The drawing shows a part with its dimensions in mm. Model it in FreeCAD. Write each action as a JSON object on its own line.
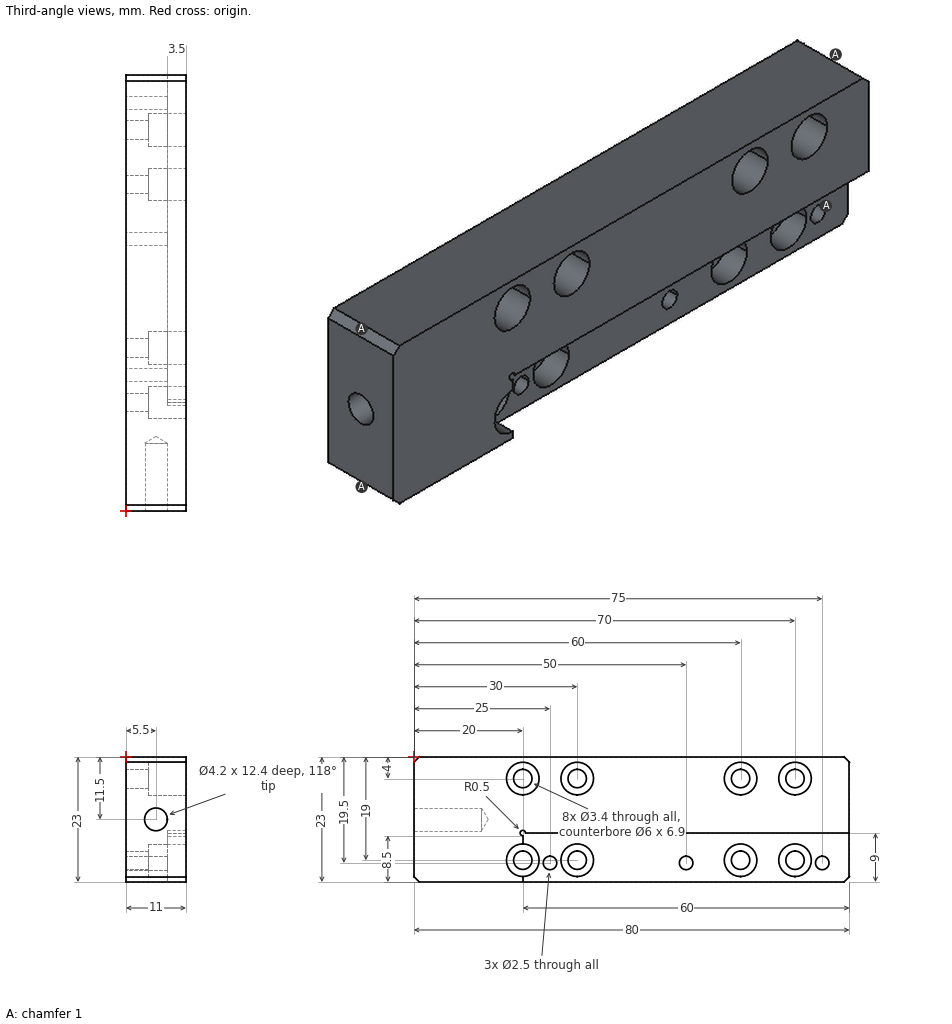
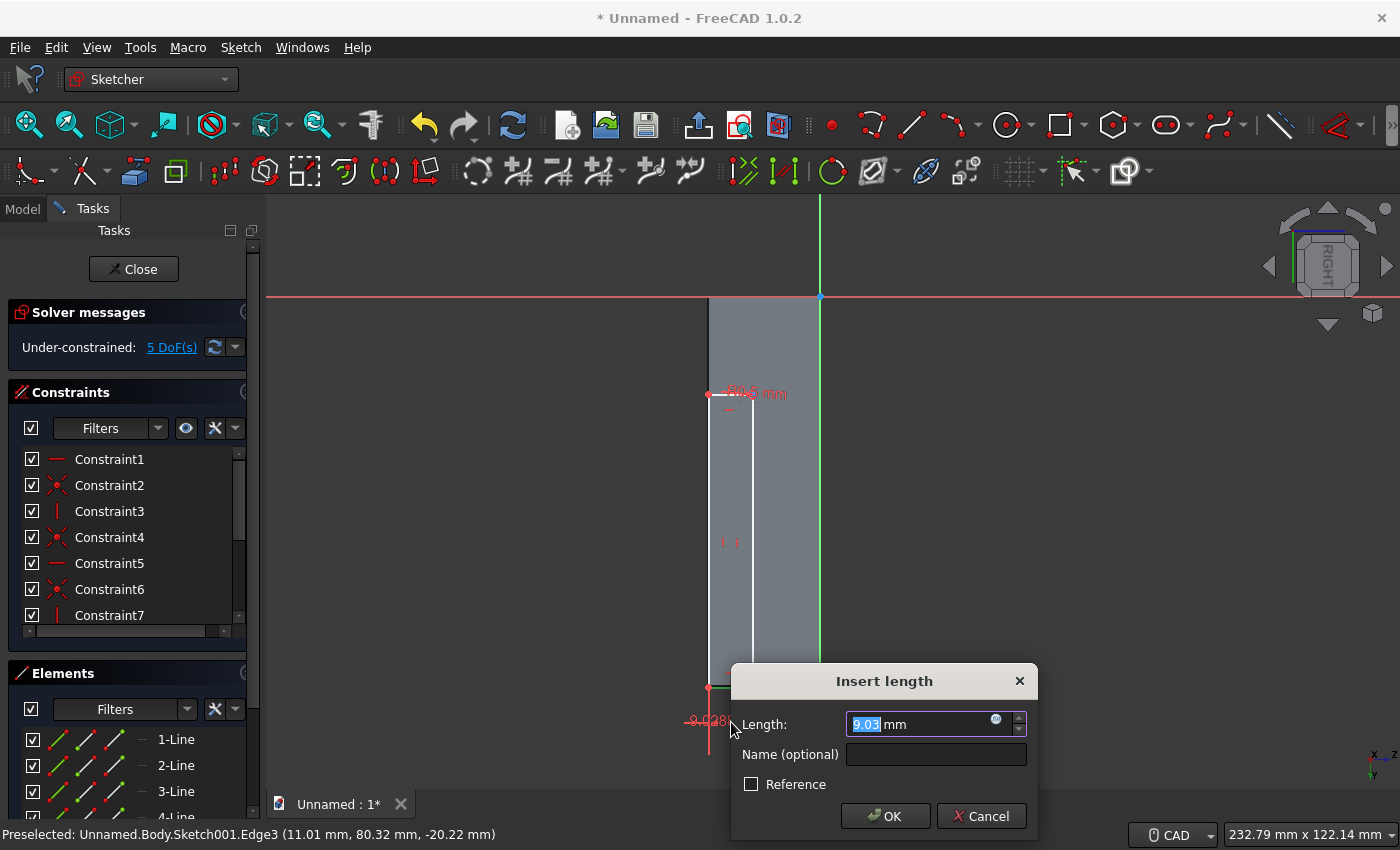
{"action": "type", "text": "9"}
{"action": "key", "text": "Return"}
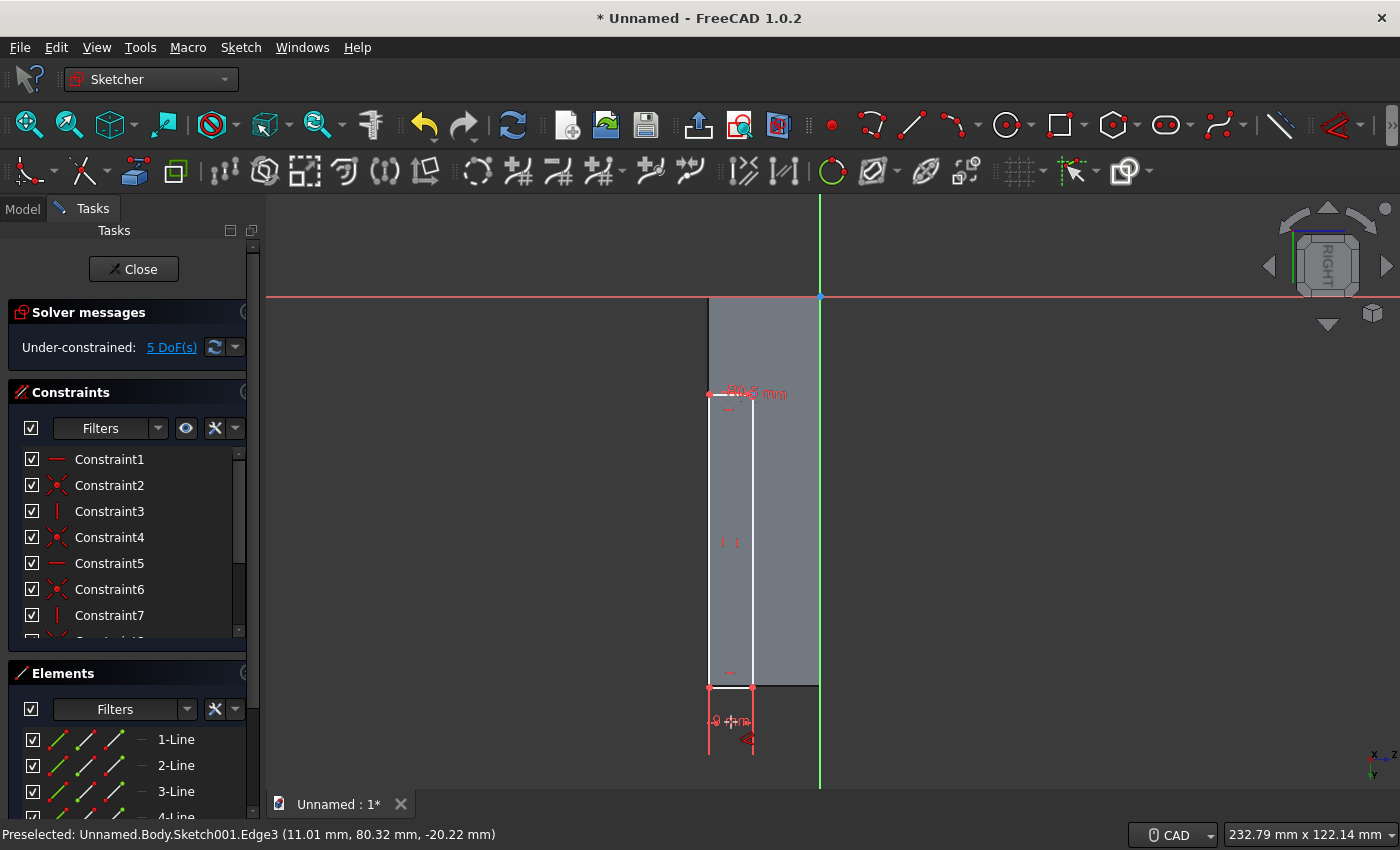
{"action": "left_click", "coordinate": [709, 483]}
{"action": "left_click", "coordinate": [675, 541]}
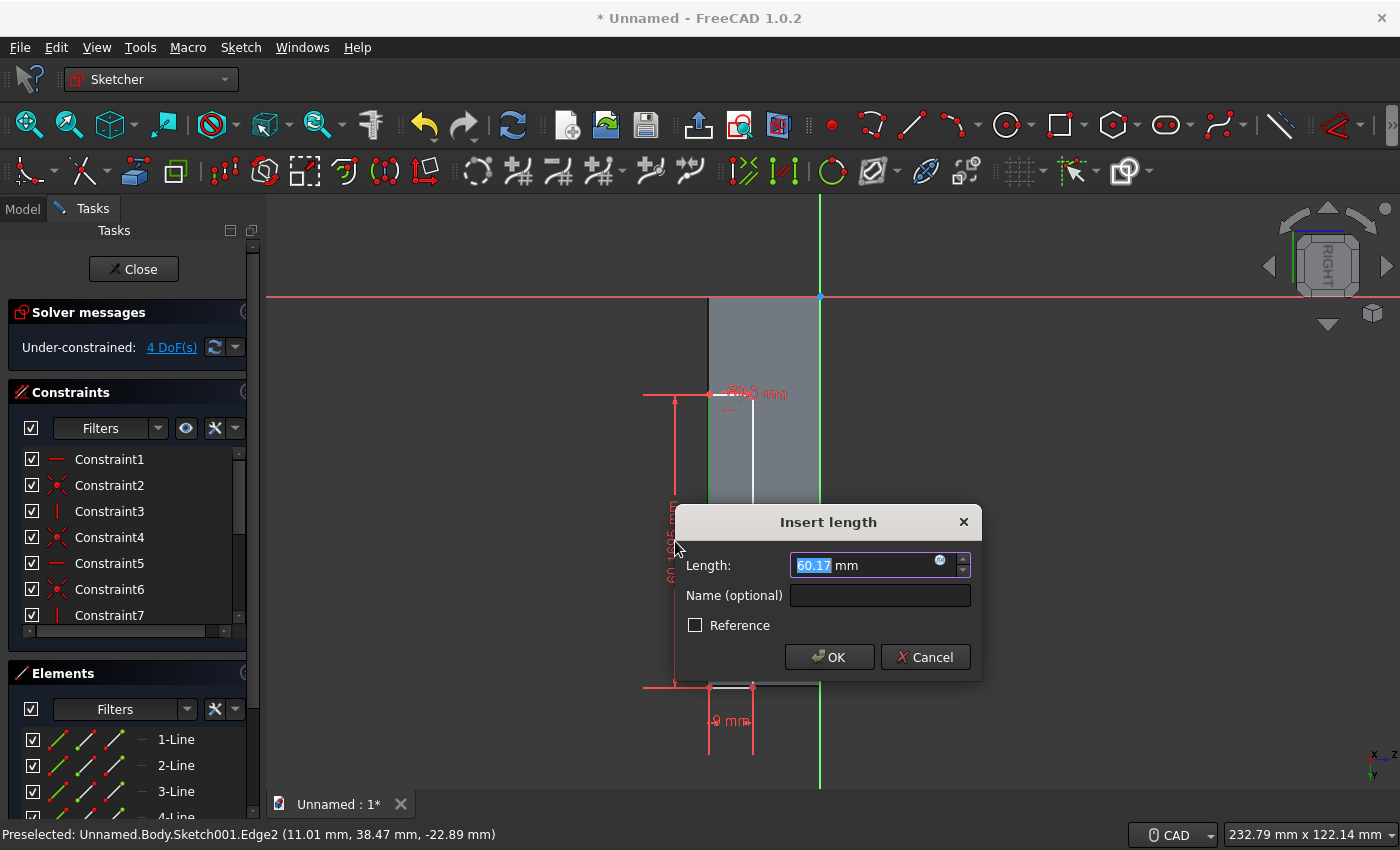
{"action": "type", "text": "60"}
{"action": "key", "text": "Return"}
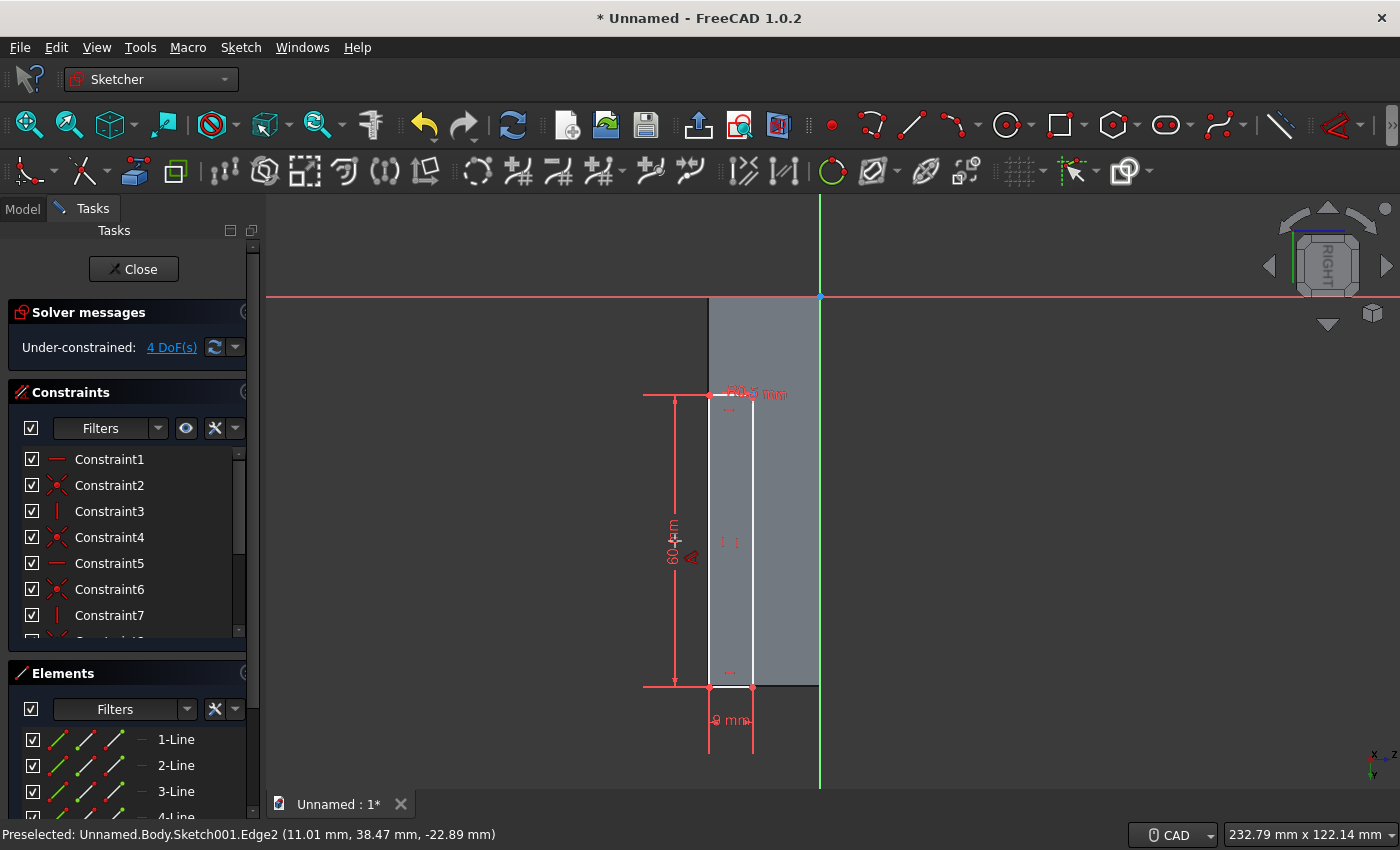
{"action": "left_click", "coordinate": [738, 395]}
{"action": "left_click", "coordinate": [730, 361]}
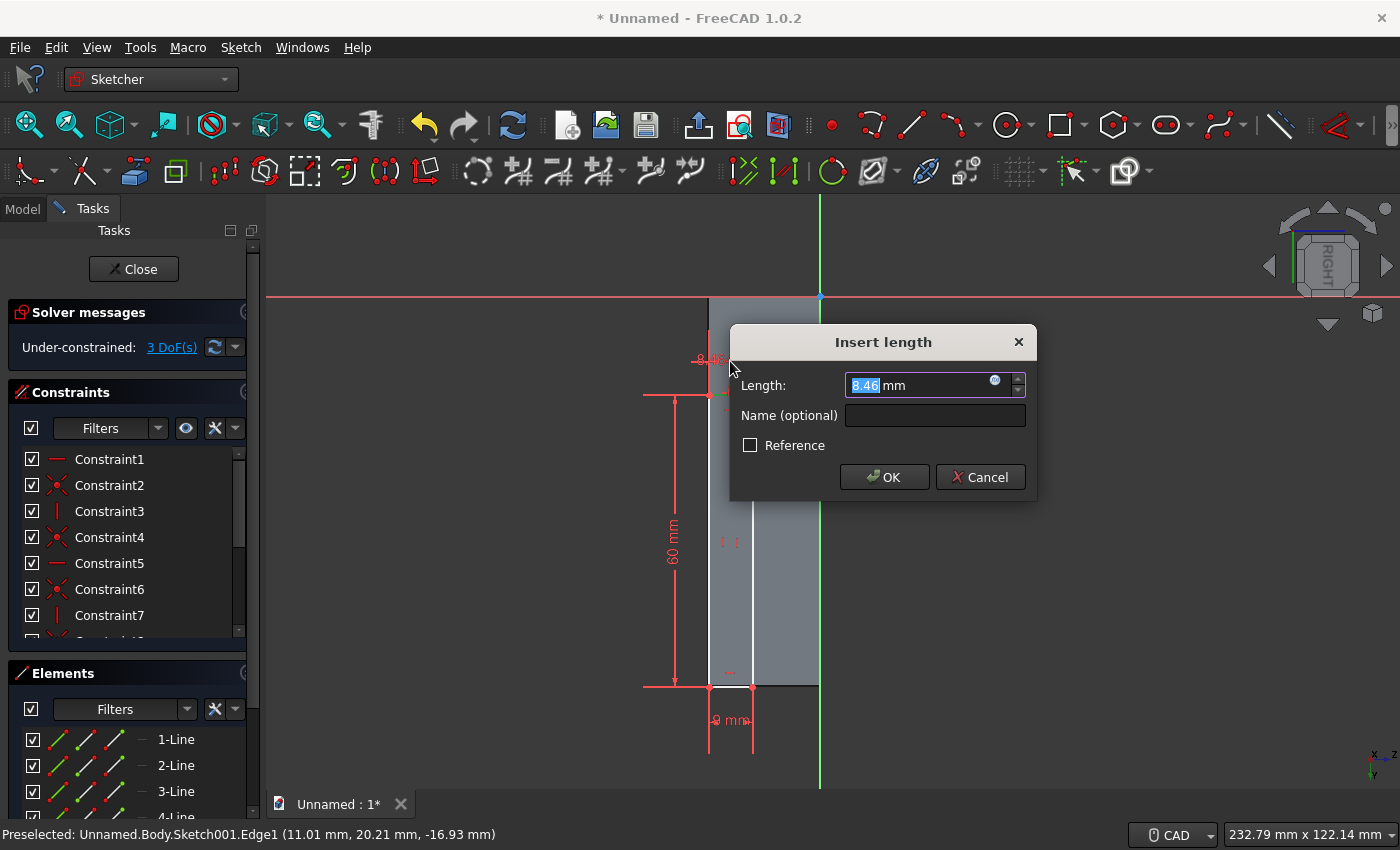
{"action": "type", "text": "8.5"}
{"action": "key", "text": "Return"}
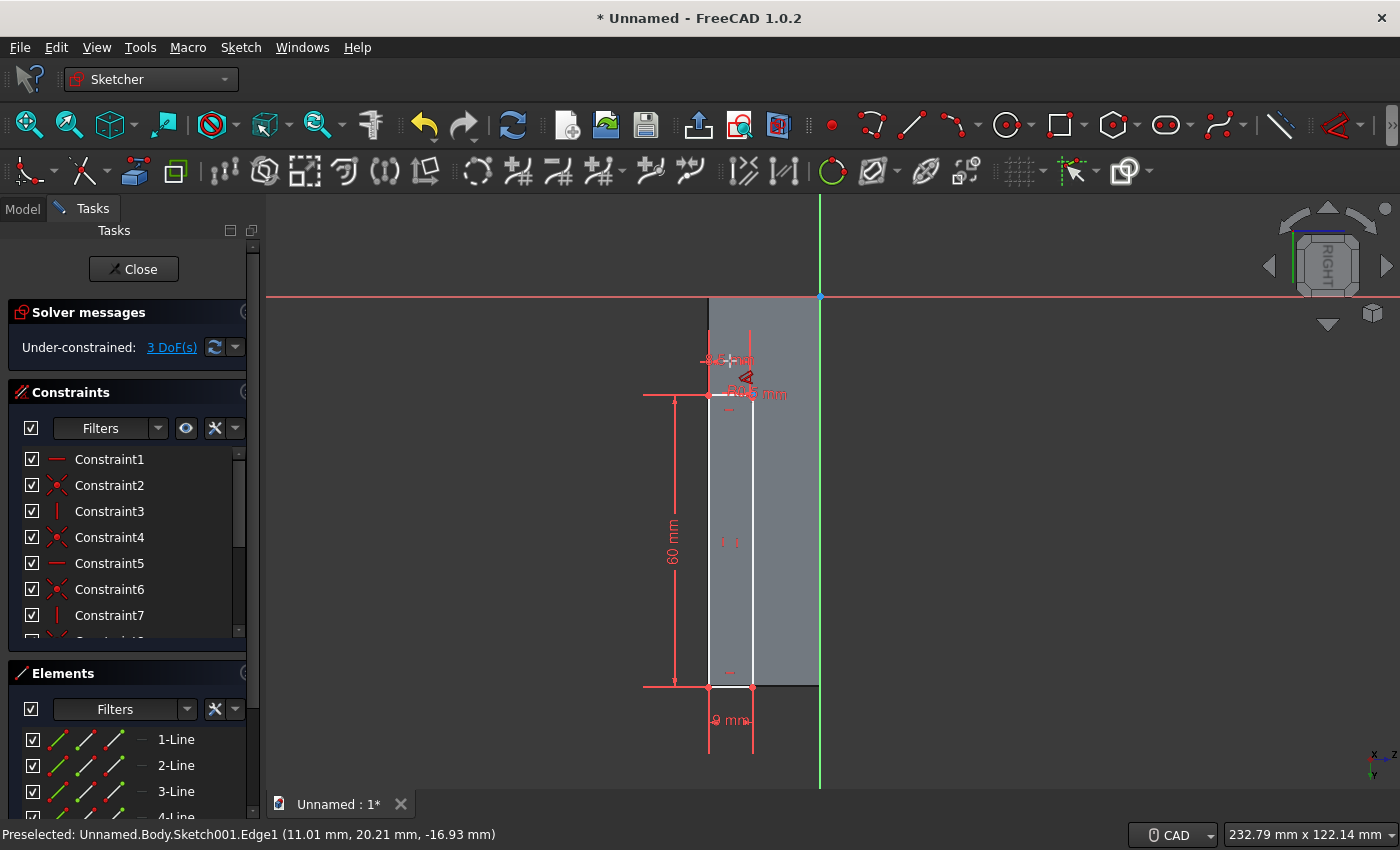
{"action": "scroll", "coordinate": [750, 395], "scroll_direction": "up", "scroll_amount": 9}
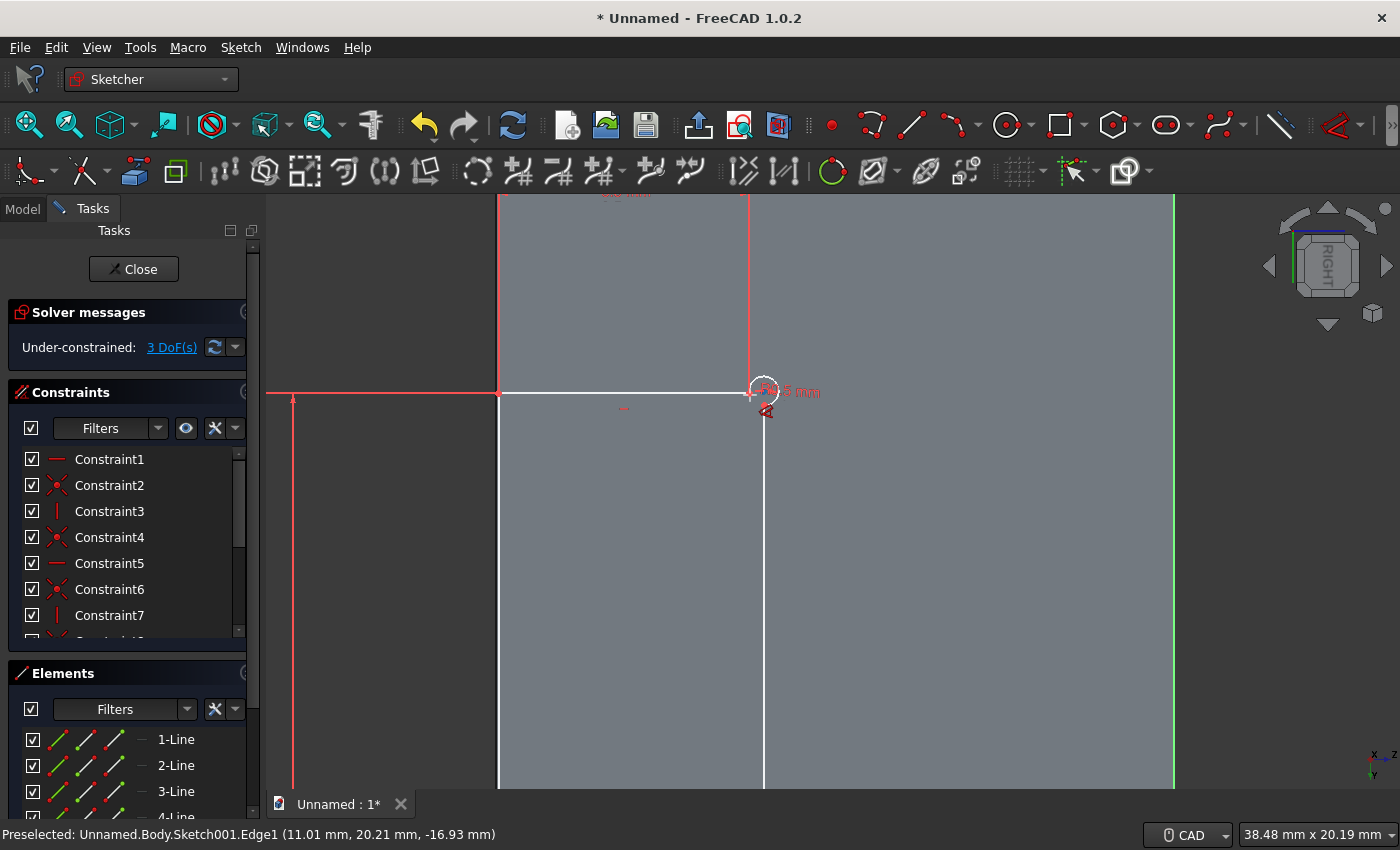
{"action": "left_click", "coordinate": [749, 393]}
{"action": "left_click", "coordinate": [1208, 308]}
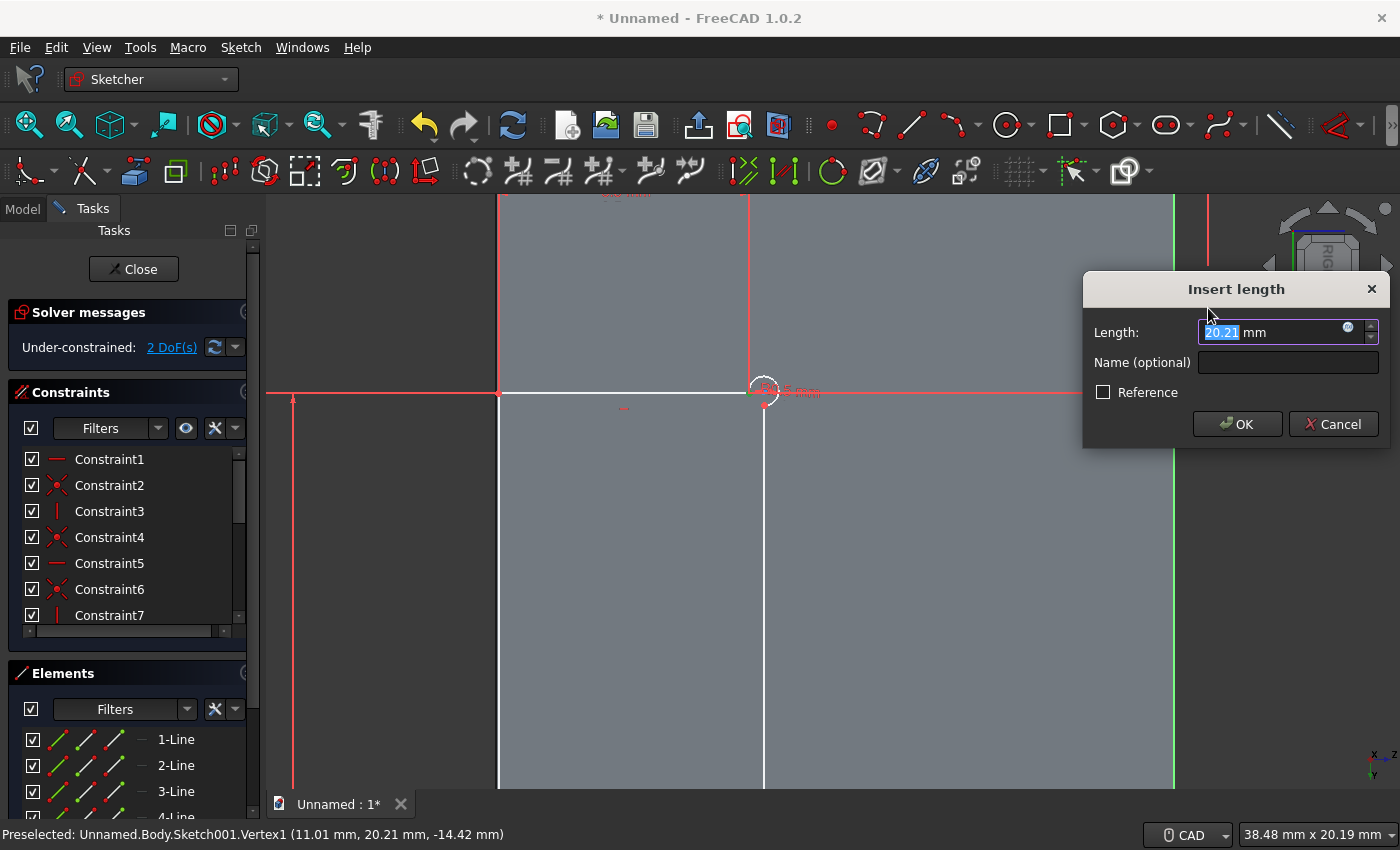
{"action": "type", "text": "20"}
{"action": "key", "text": "Return"}